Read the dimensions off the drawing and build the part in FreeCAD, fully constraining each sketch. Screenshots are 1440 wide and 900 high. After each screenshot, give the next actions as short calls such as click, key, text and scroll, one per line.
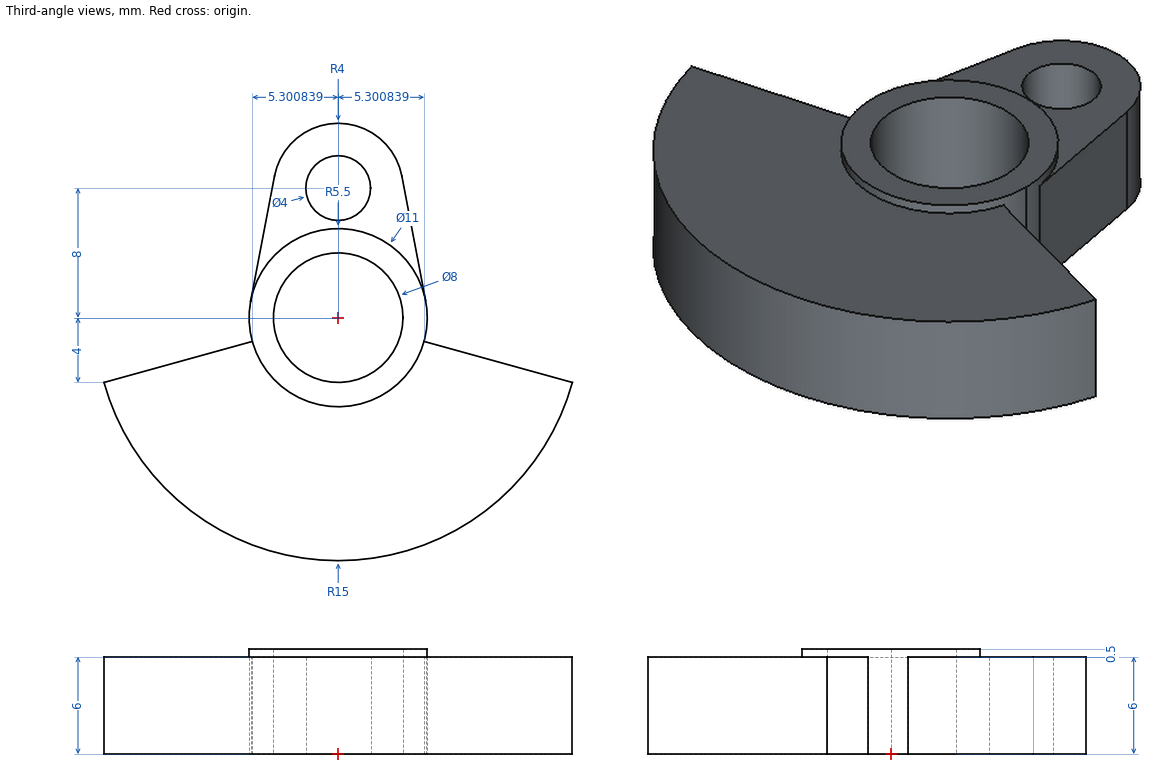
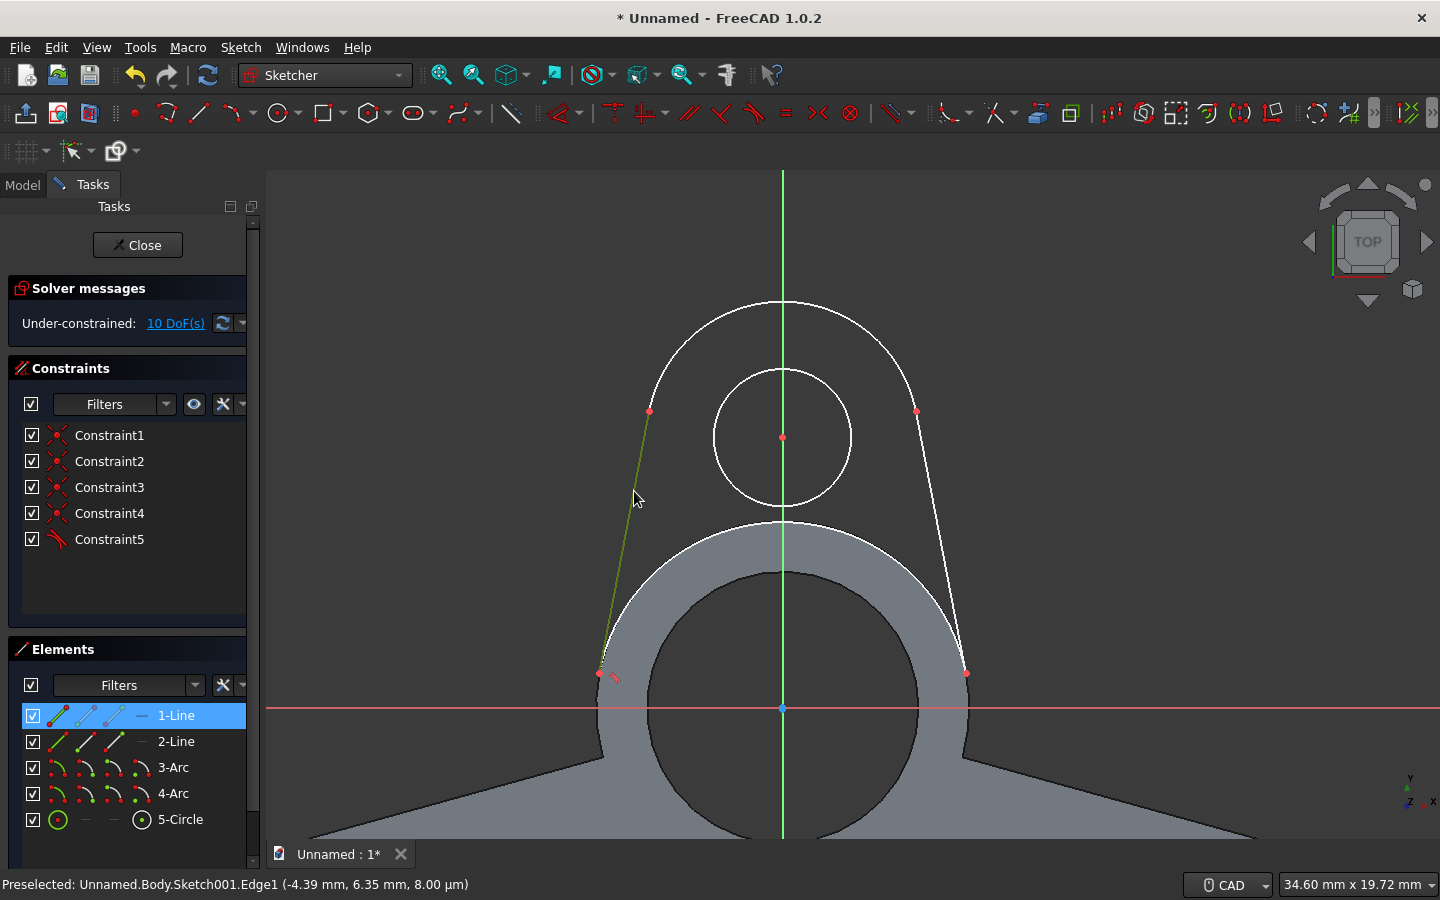
click(854, 322)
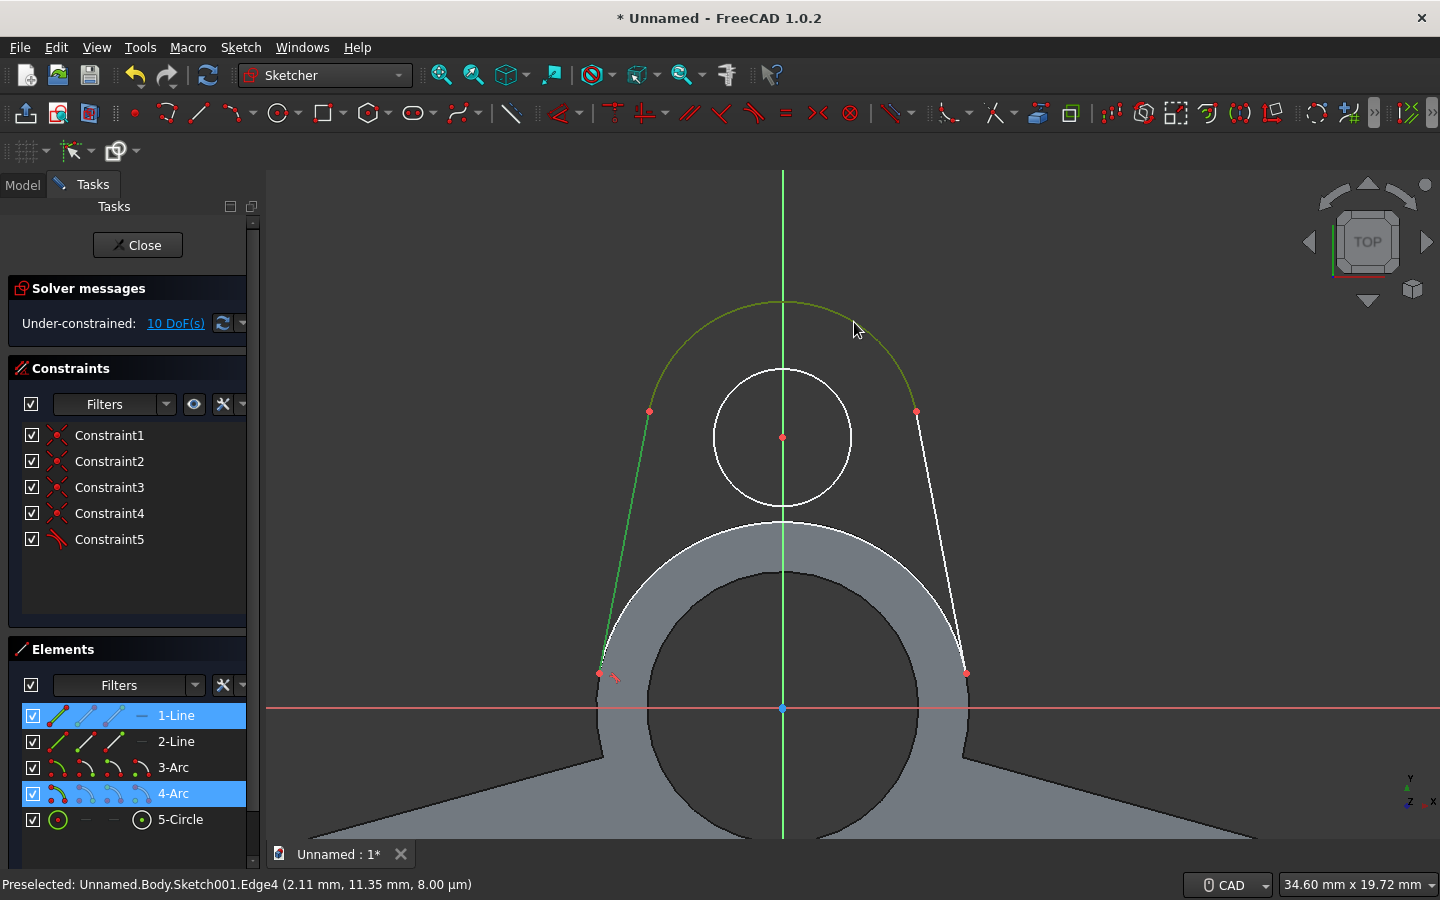
key(t)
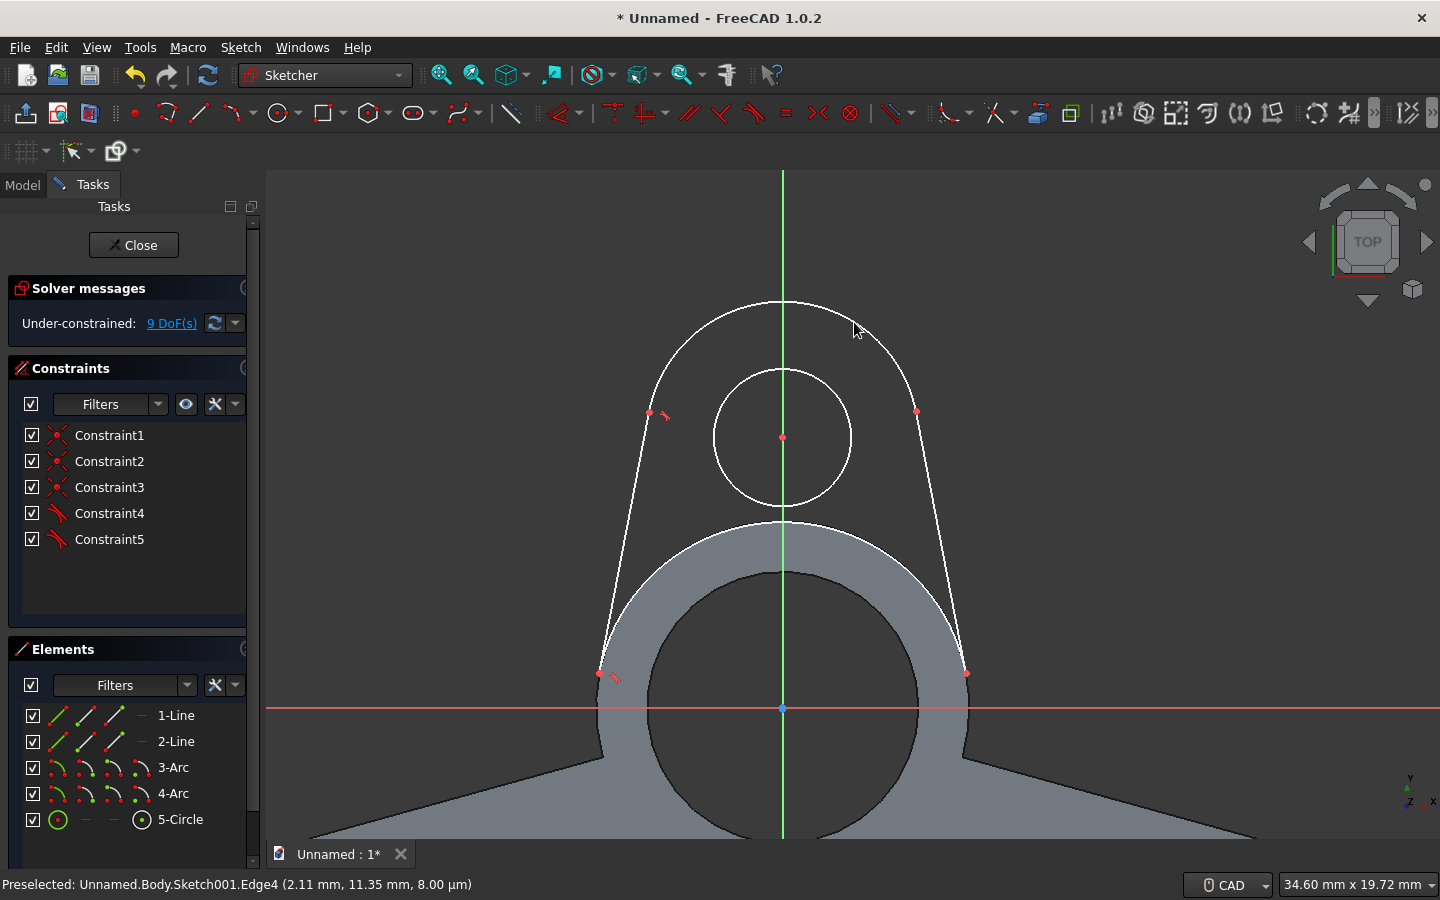
click(951, 595)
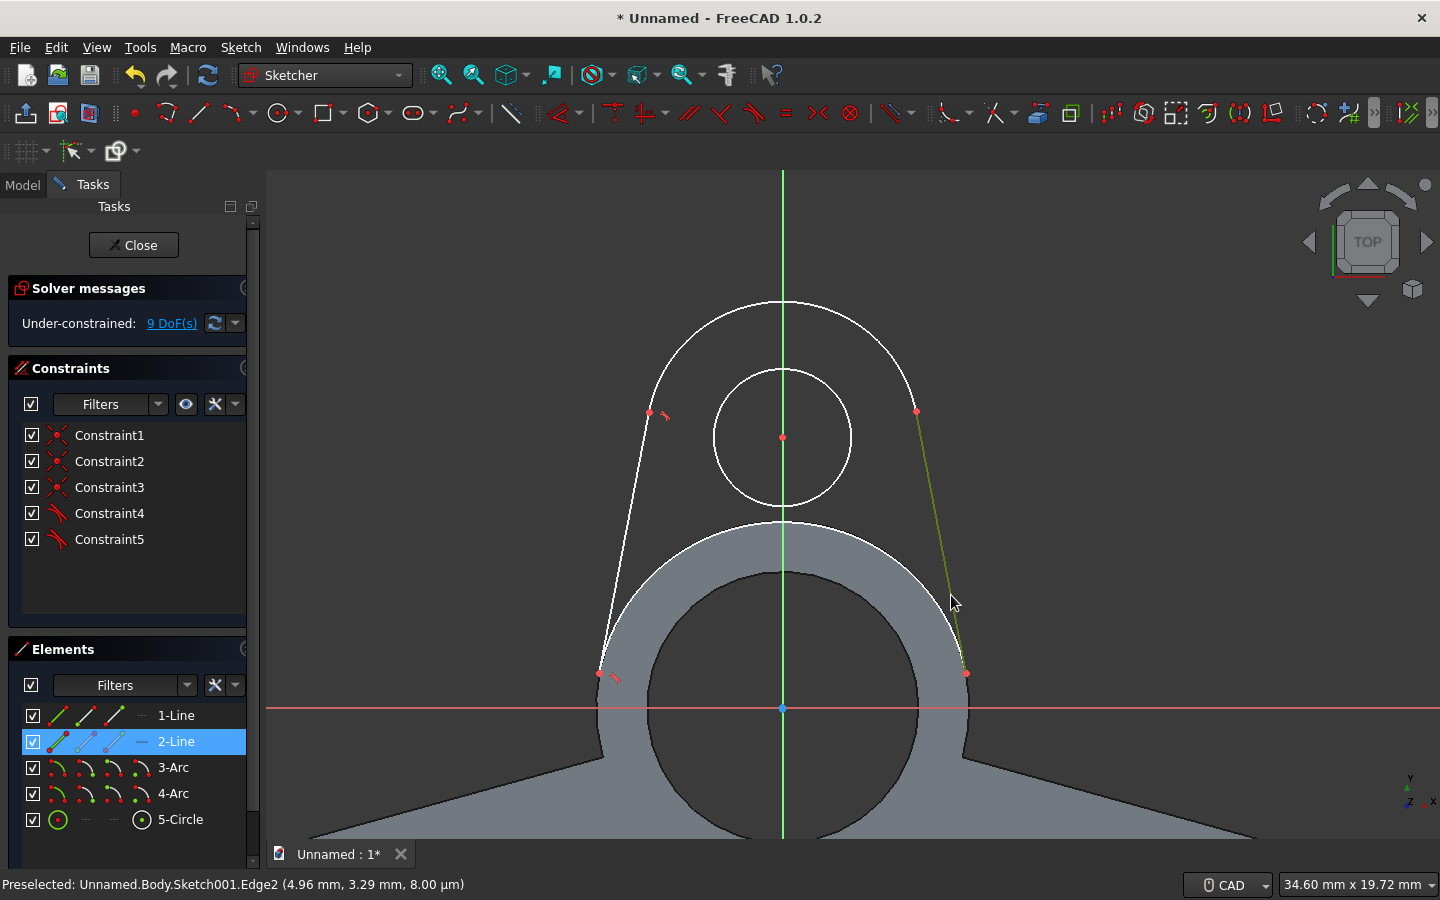
click(881, 550)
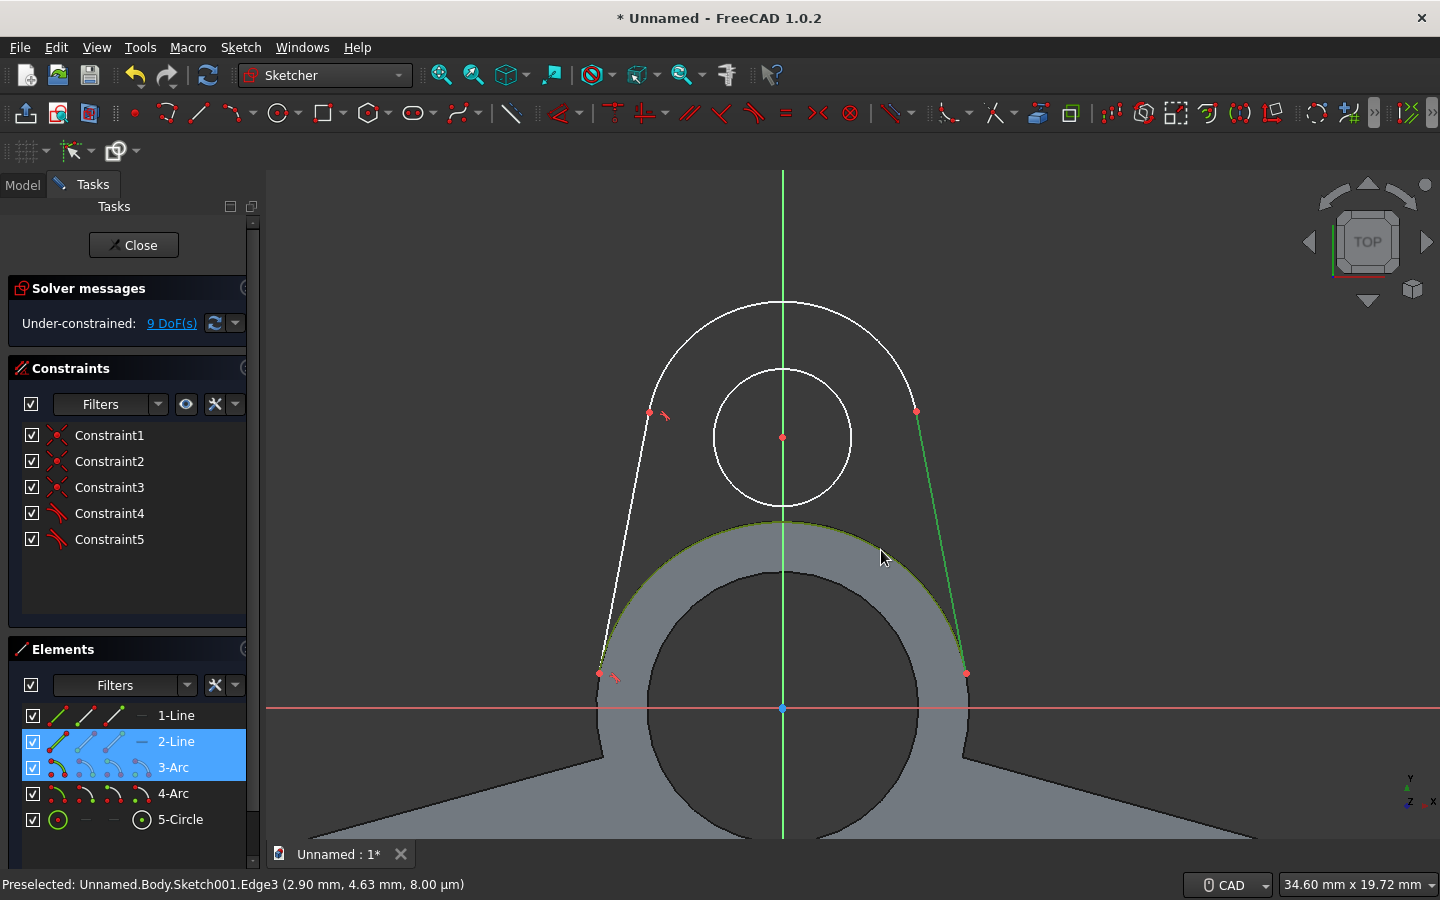
click(754, 114)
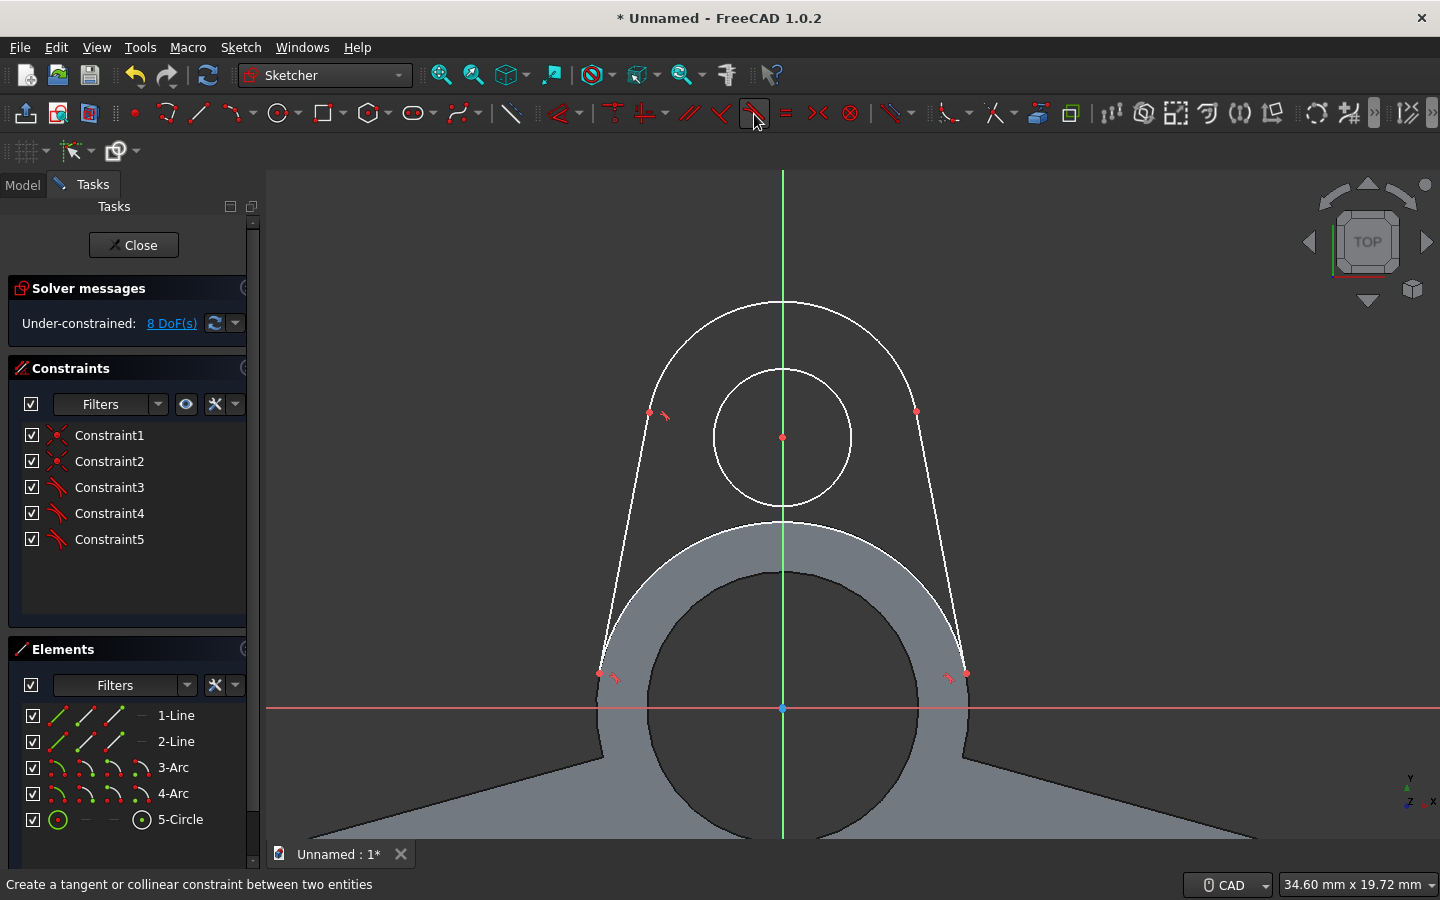
click(951, 595)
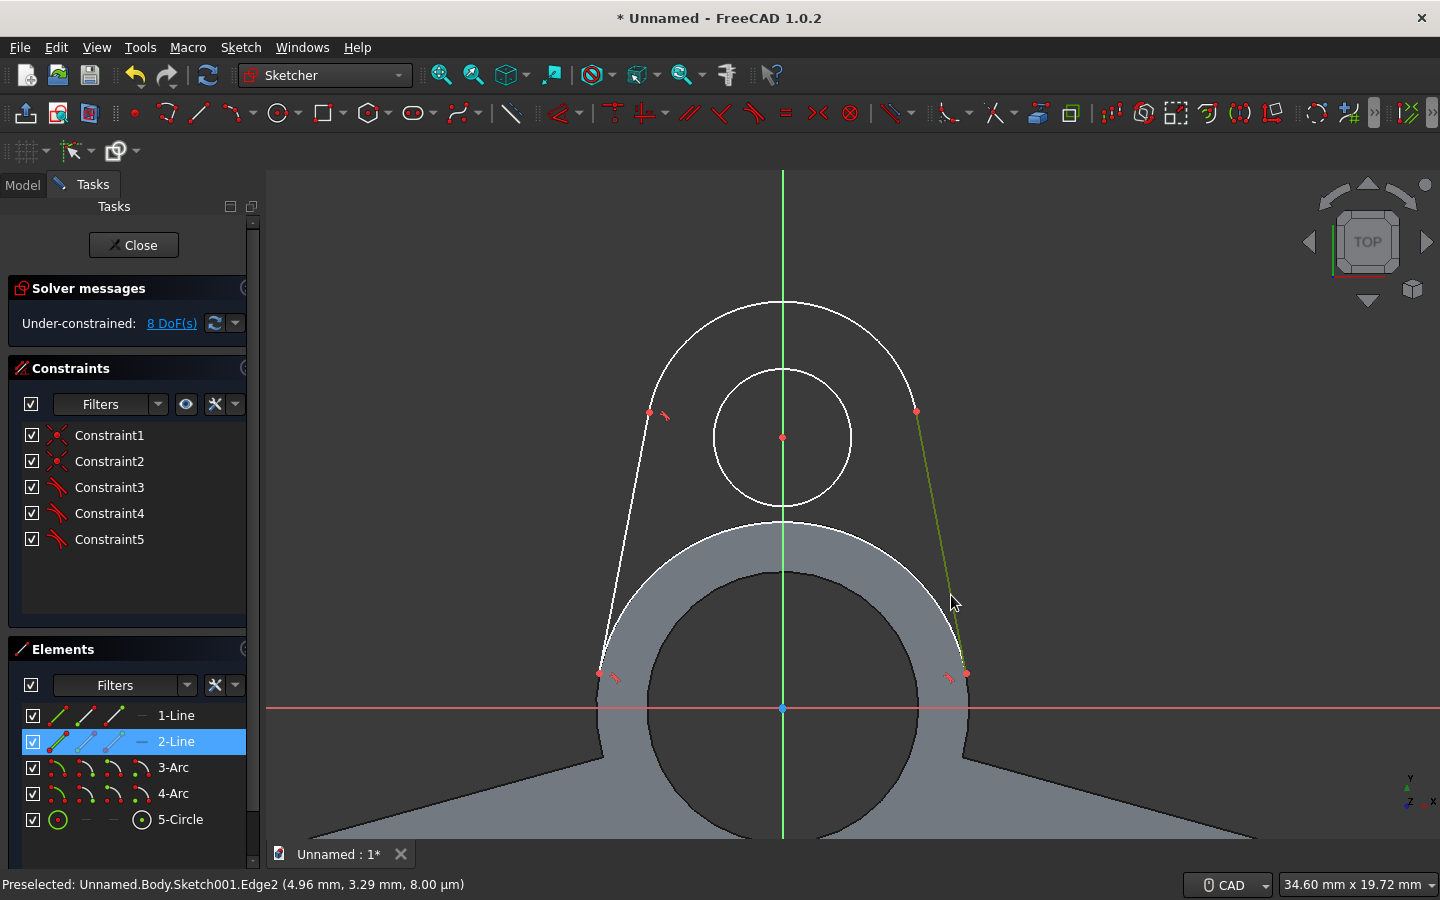
click(854, 322)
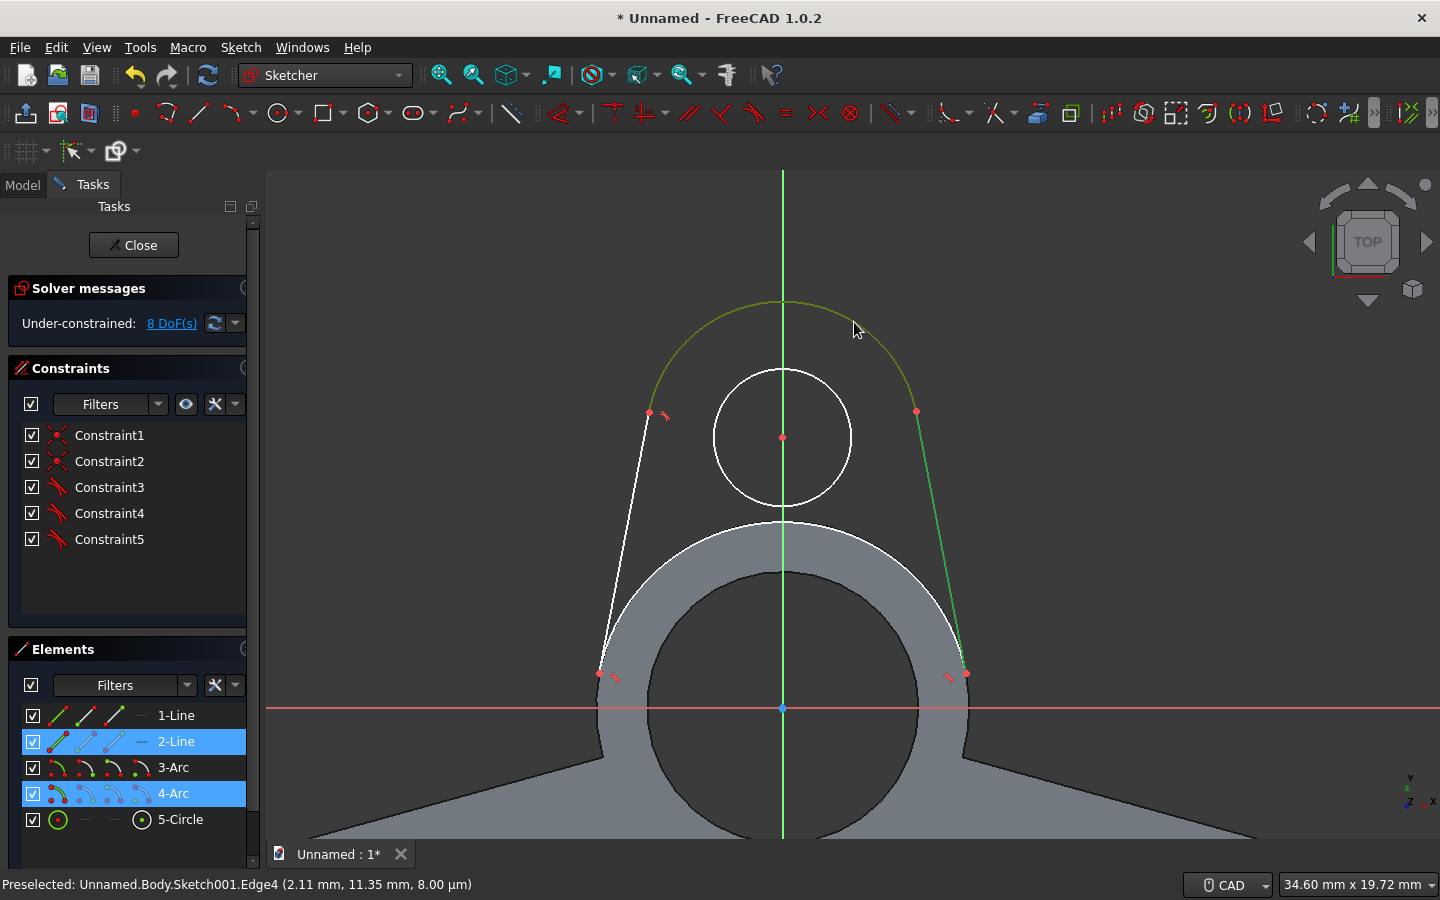
key(t)